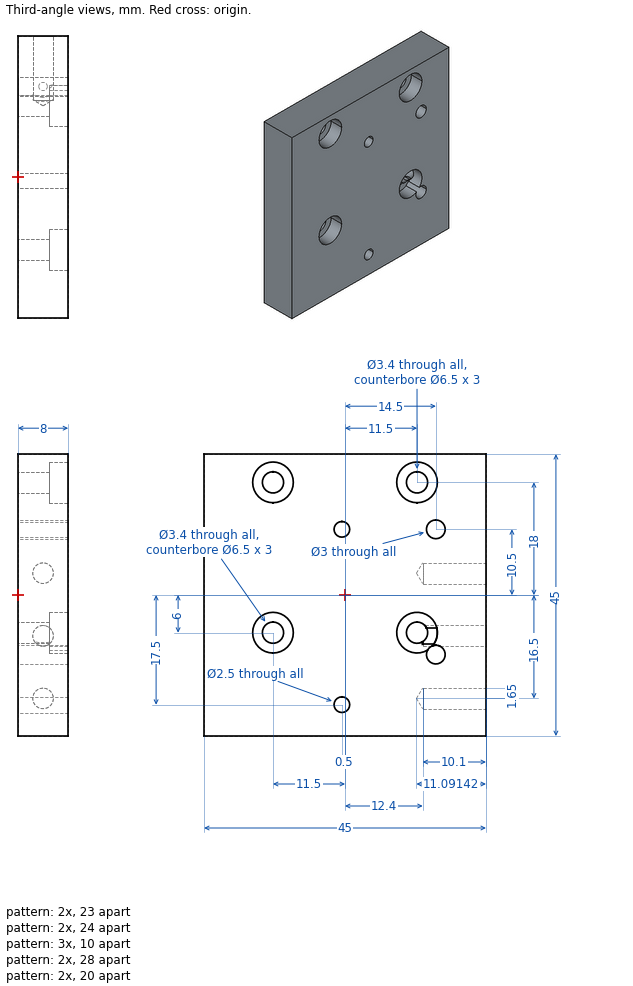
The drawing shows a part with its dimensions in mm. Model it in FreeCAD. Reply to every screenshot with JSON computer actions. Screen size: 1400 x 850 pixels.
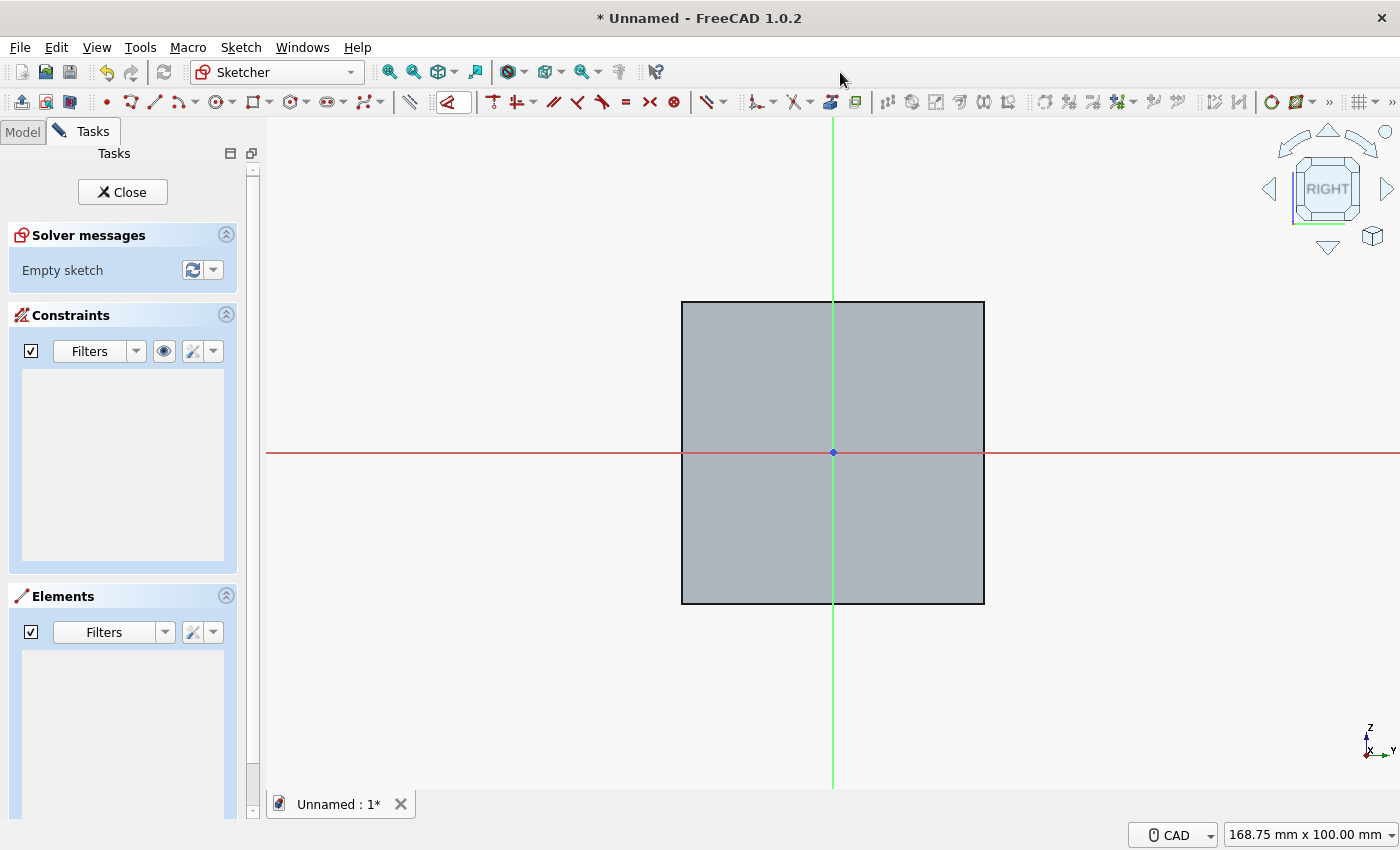
{"action": "scroll", "coordinate": [918, 326], "scroll_direction": "up", "scroll_amount": 15}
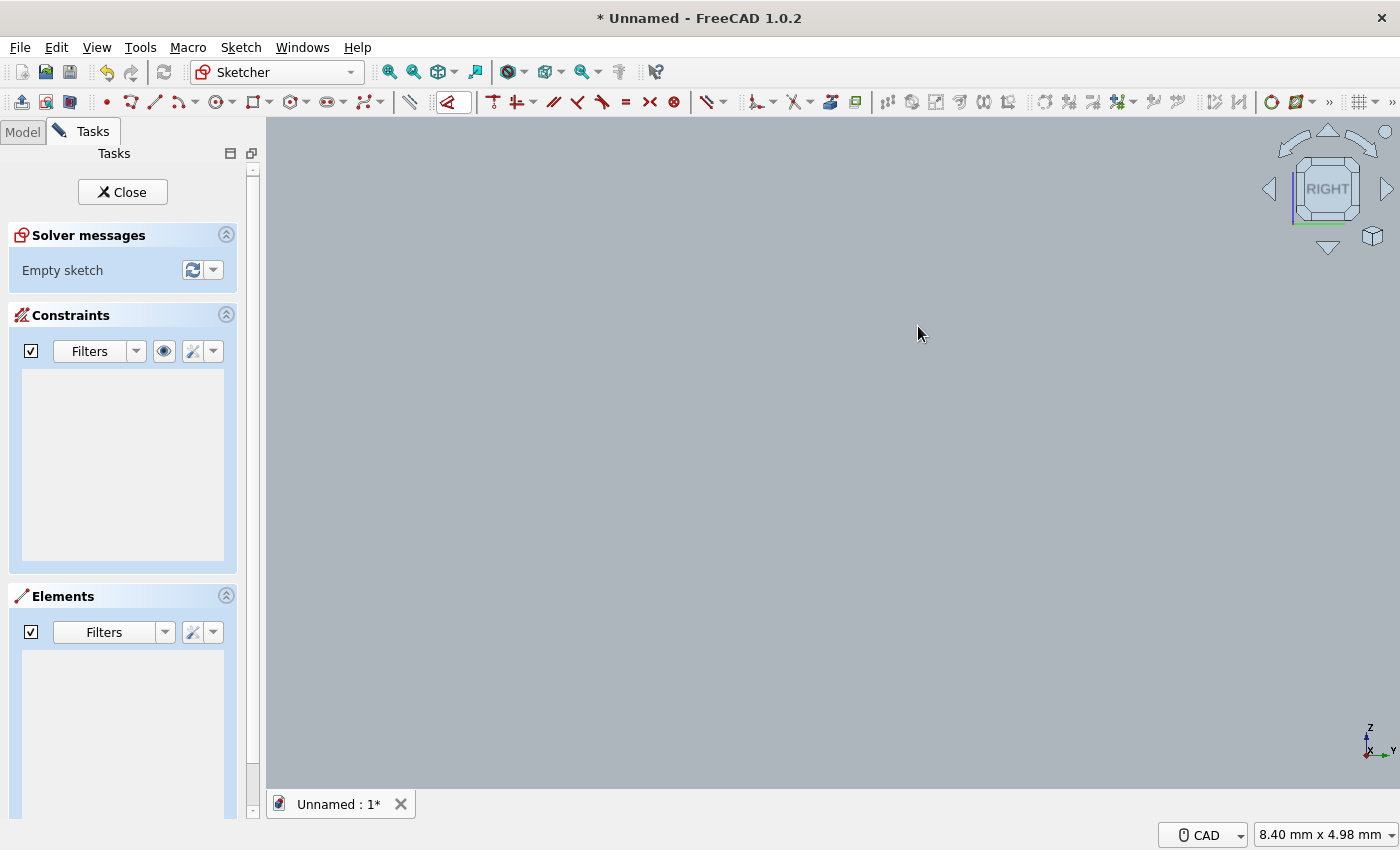
{"action": "left_click", "coordinate": [216, 102]}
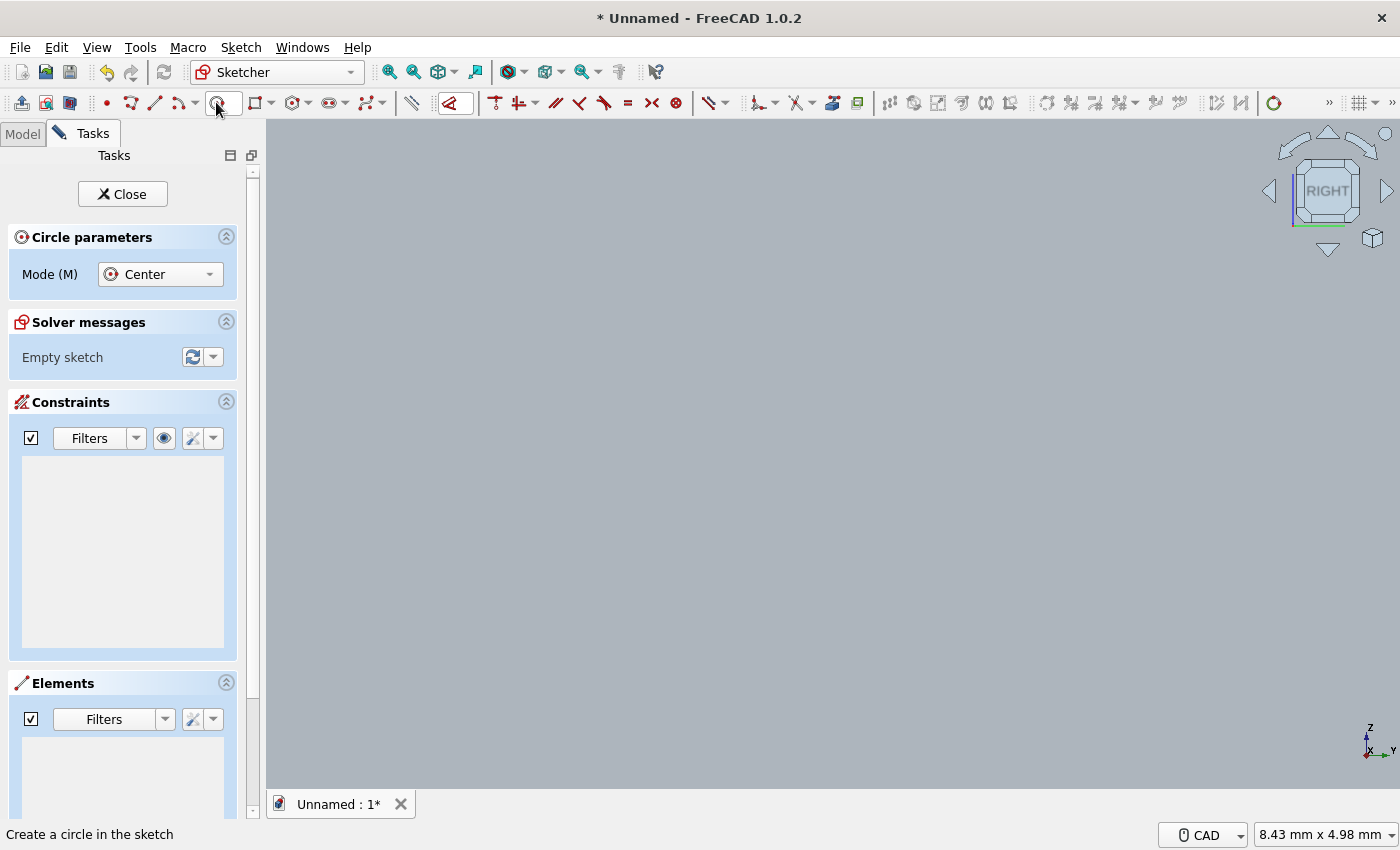
{"action": "left_click", "coordinate": [752, 442]}
{"action": "left_click", "coordinate": [914, 281]}
{"action": "key", "text": "Escape"}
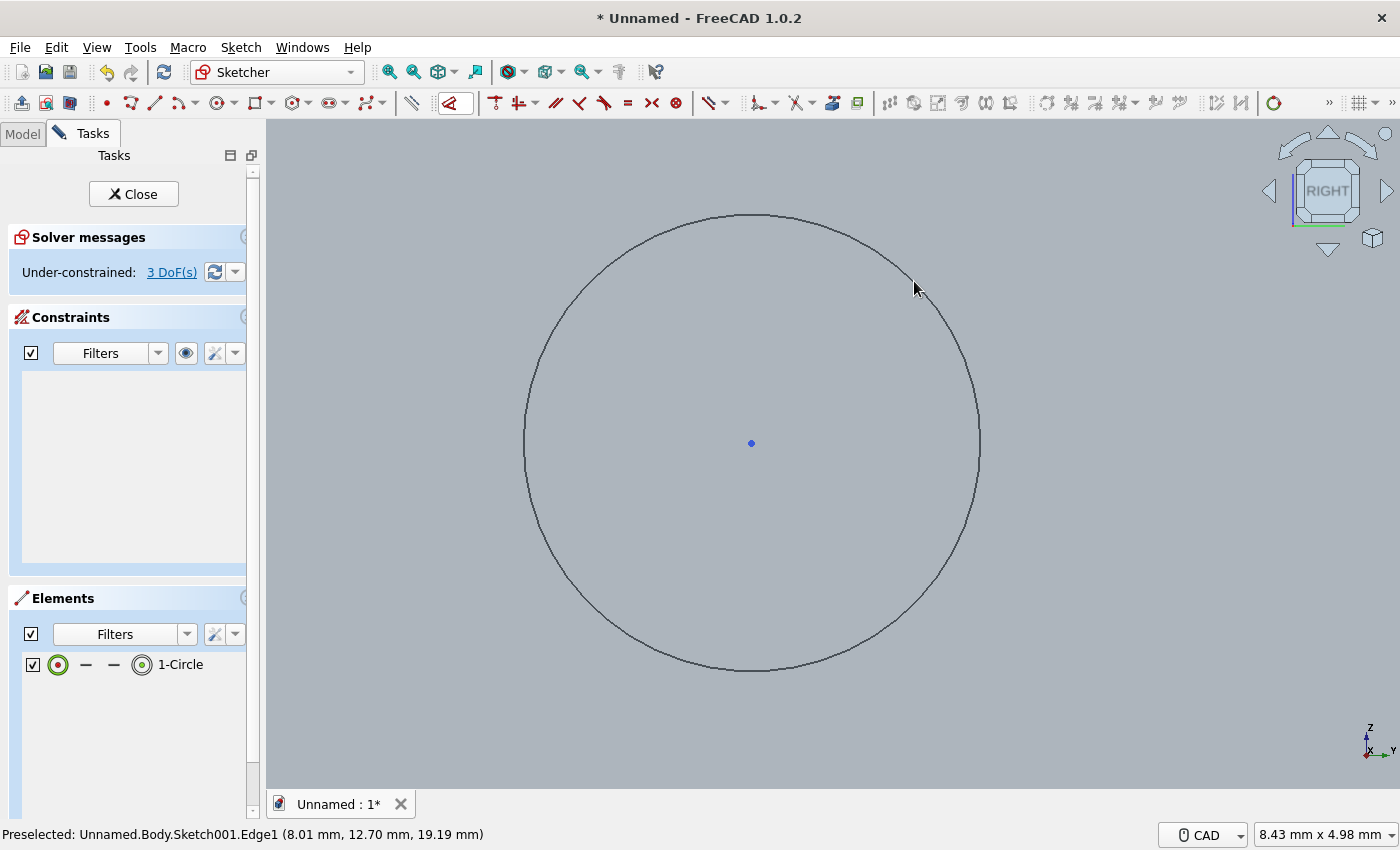
{"action": "key", "text": "d"}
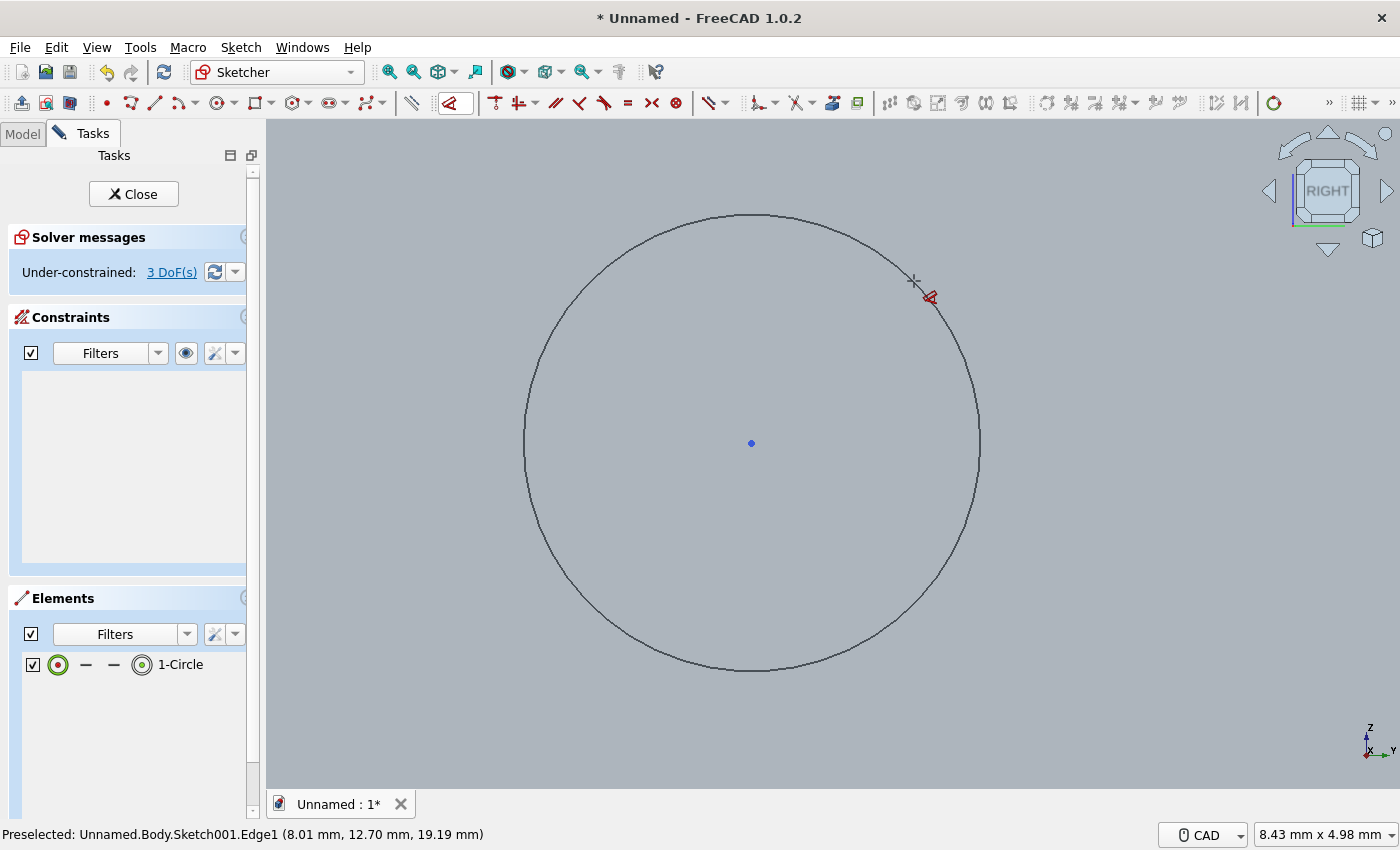
{"action": "left_click", "coordinate": [913, 281]}
{"action": "left_click", "coordinate": [936, 258]}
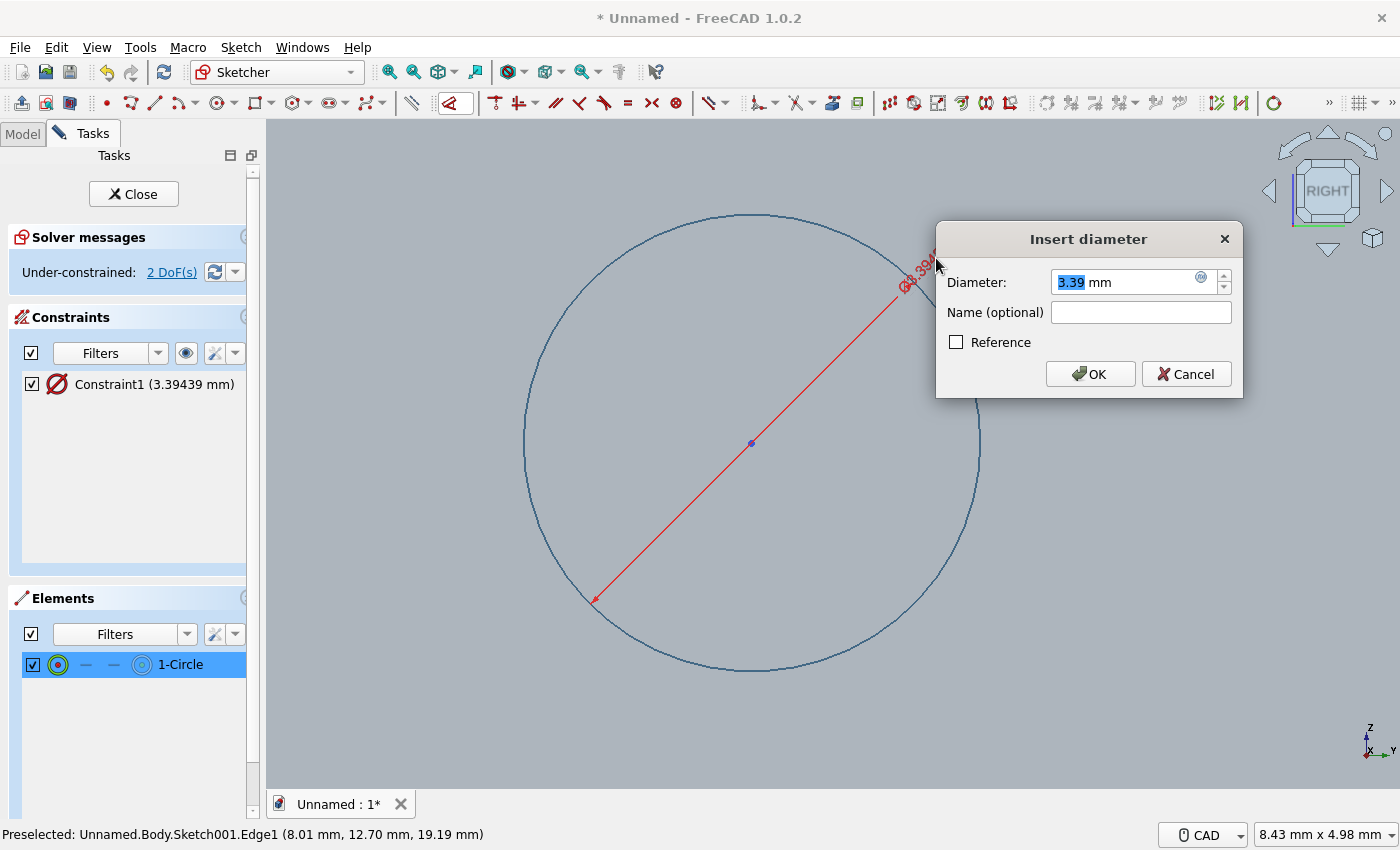
{"action": "type", "text": "3.4"}
{"action": "key", "text": "Return"}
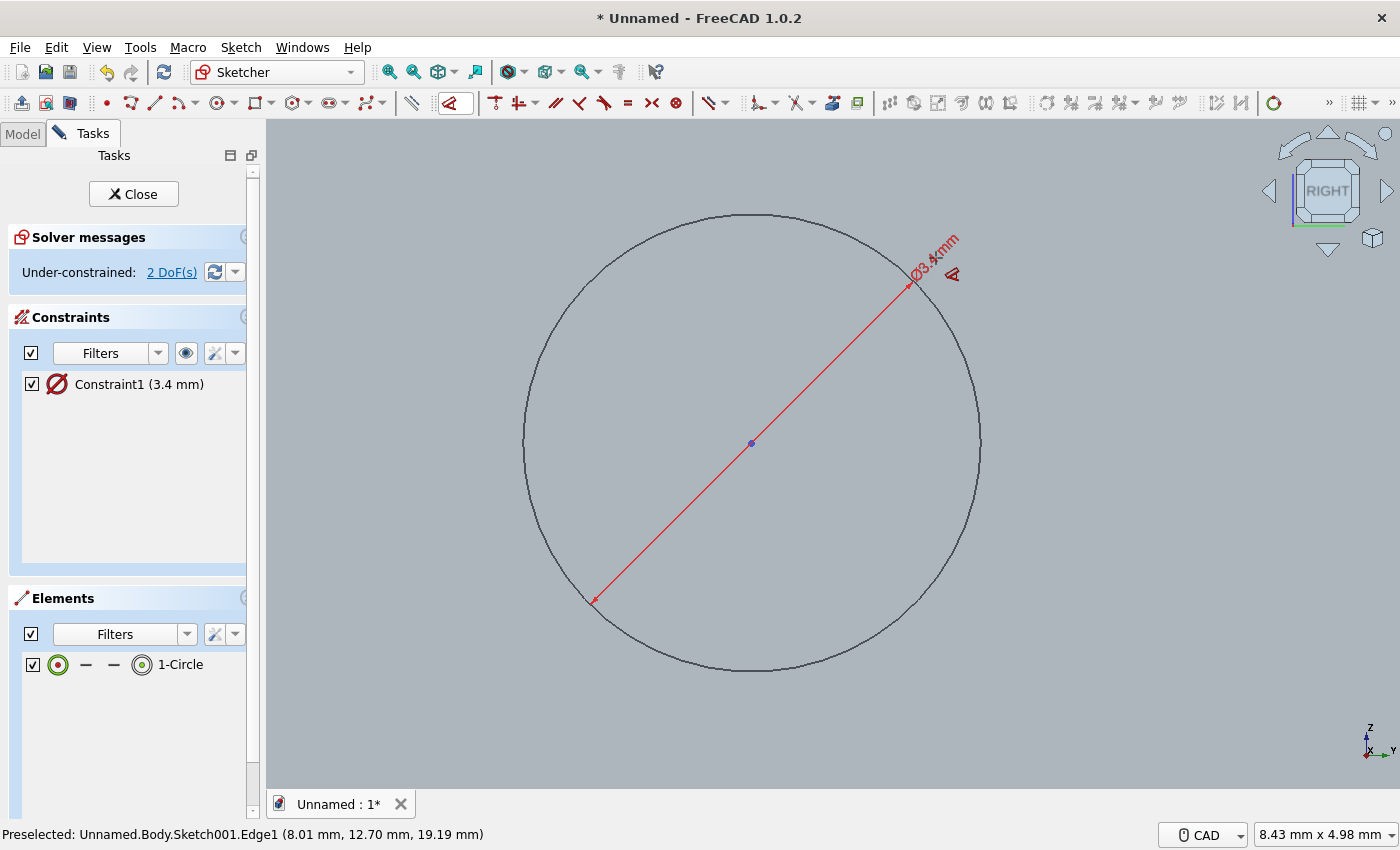
{"action": "left_click", "coordinate": [752, 443]}
{"action": "left_click", "coordinate": [786, 602]}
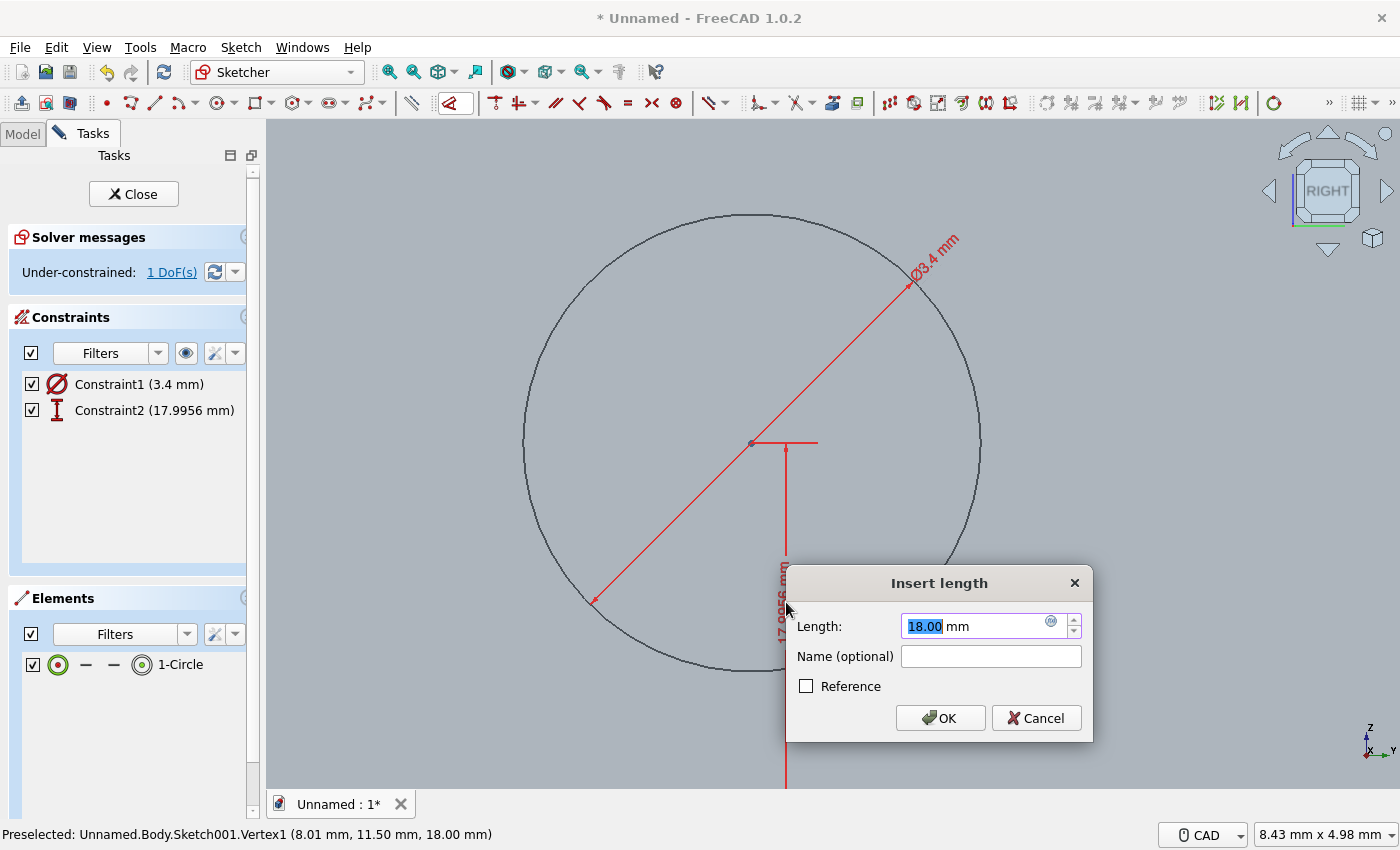
{"action": "type", "text": "18"}
{"action": "key", "text": "Return"}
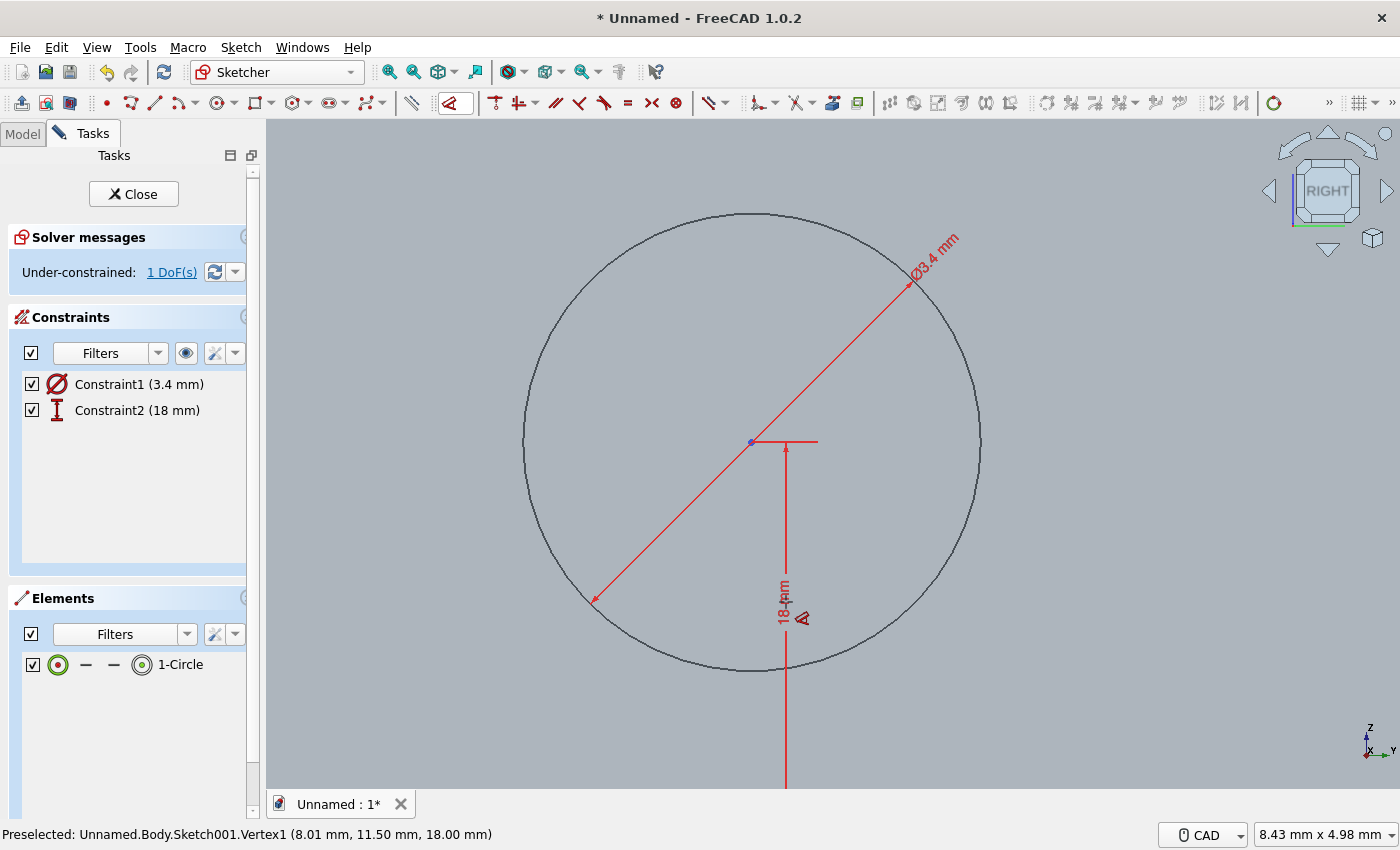
{"action": "left_click", "coordinate": [752, 442]}
{"action": "left_click", "coordinate": [418, 408]}